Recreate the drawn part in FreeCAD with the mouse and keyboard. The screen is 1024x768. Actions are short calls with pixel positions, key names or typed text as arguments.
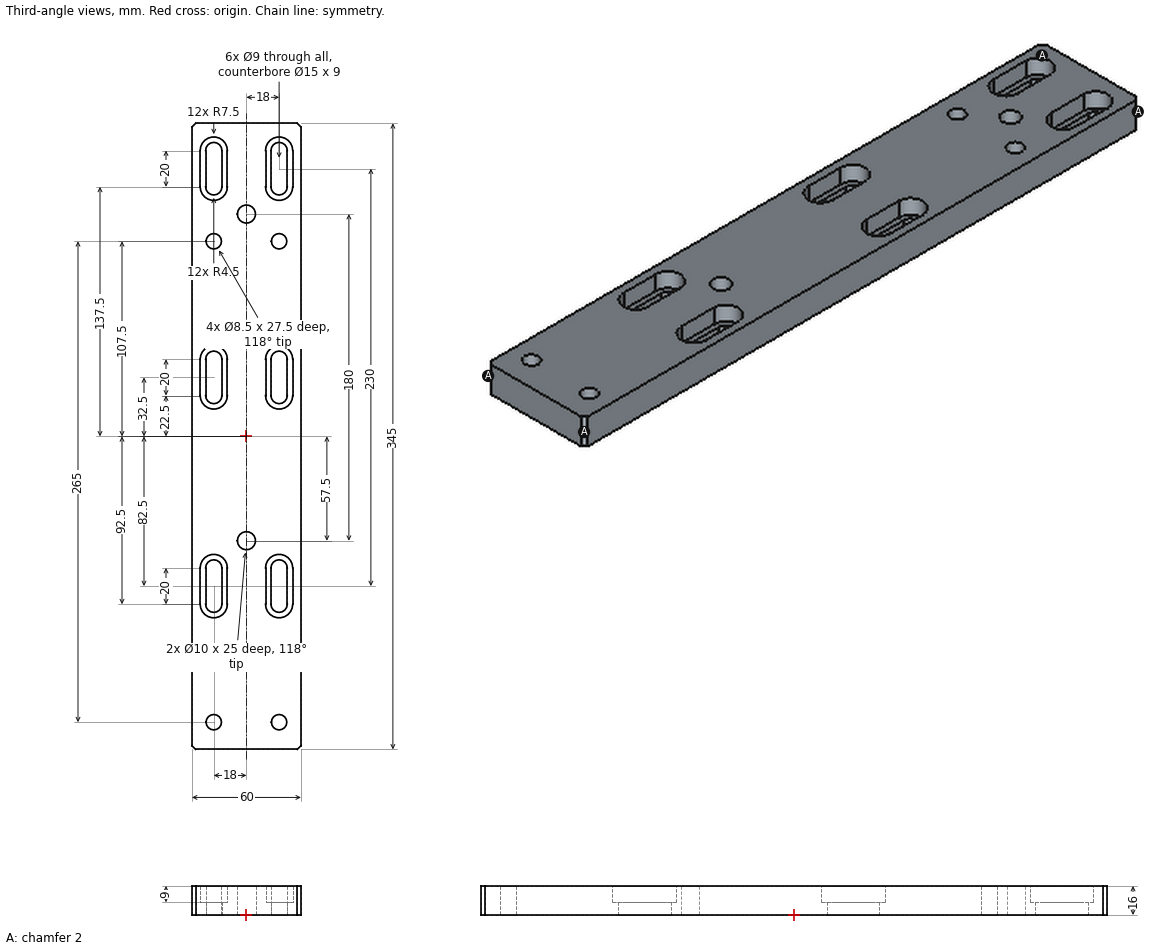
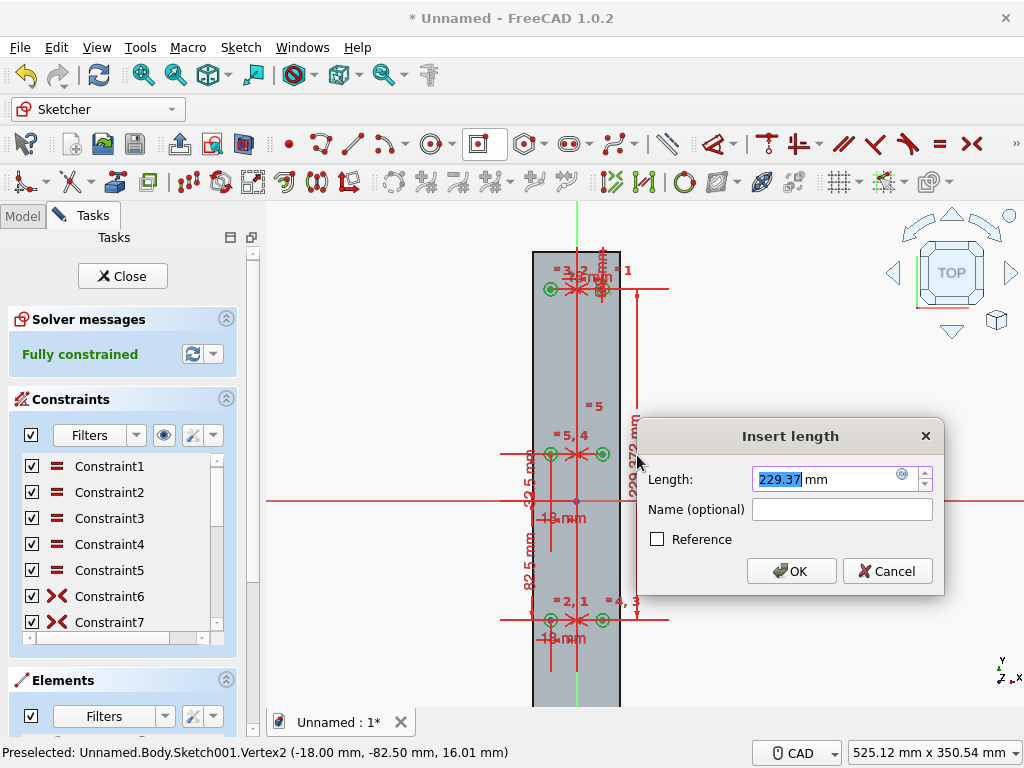
text(230)
key(Return)
key(Escape)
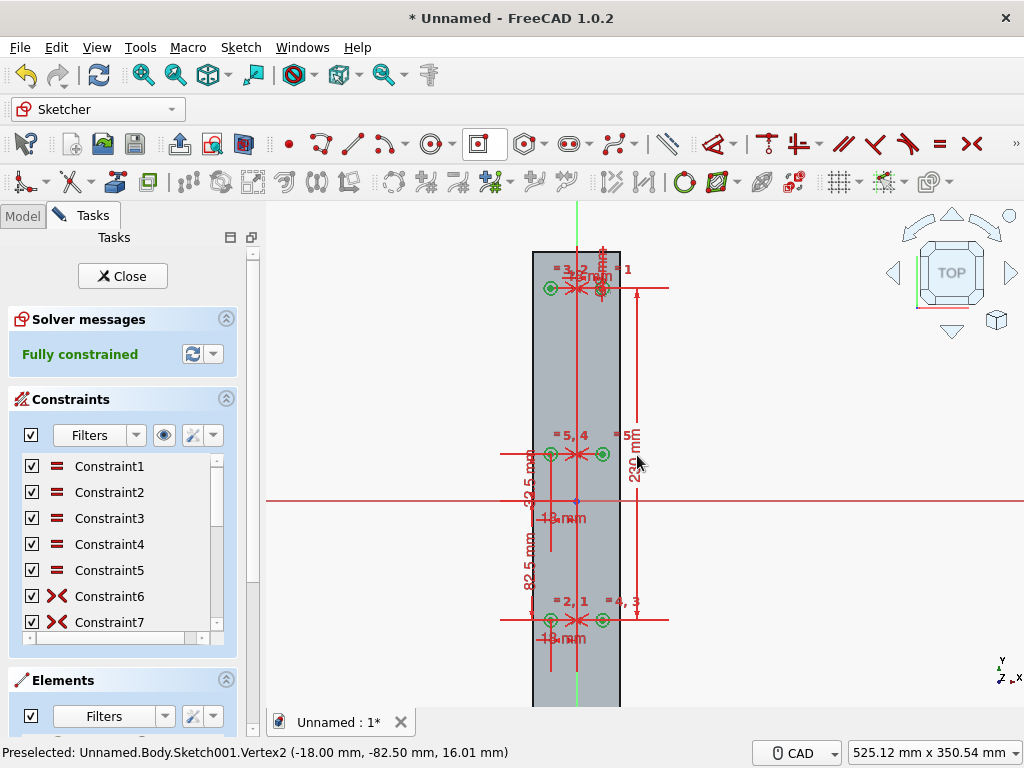
click(123, 276)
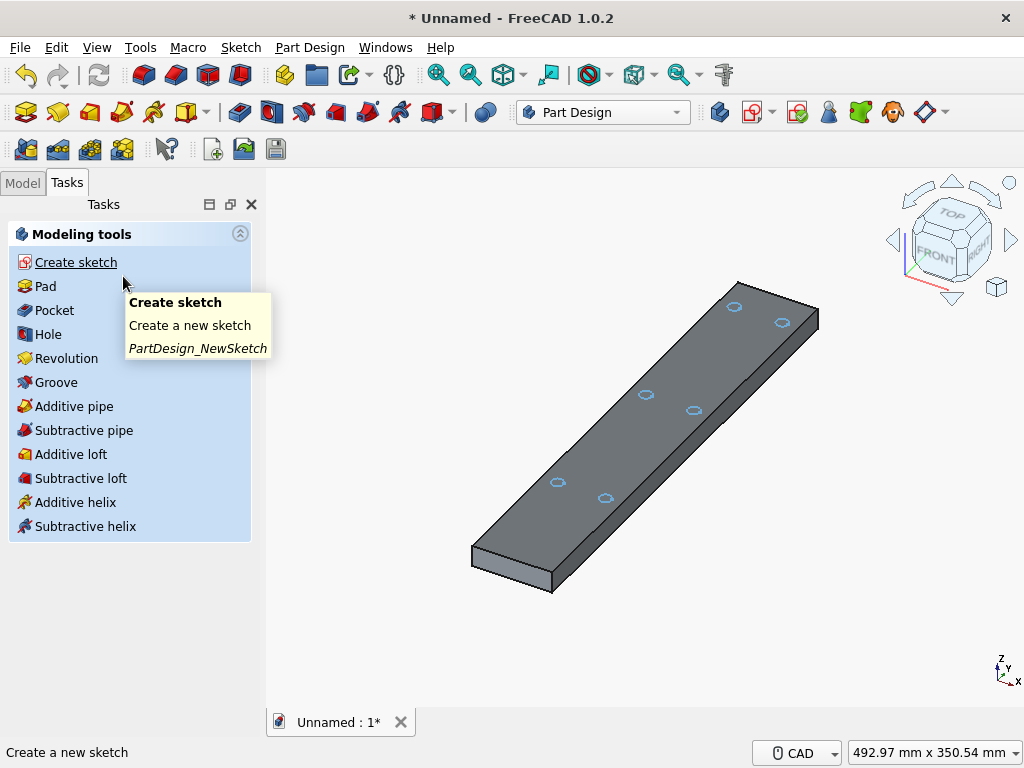
click(272, 112)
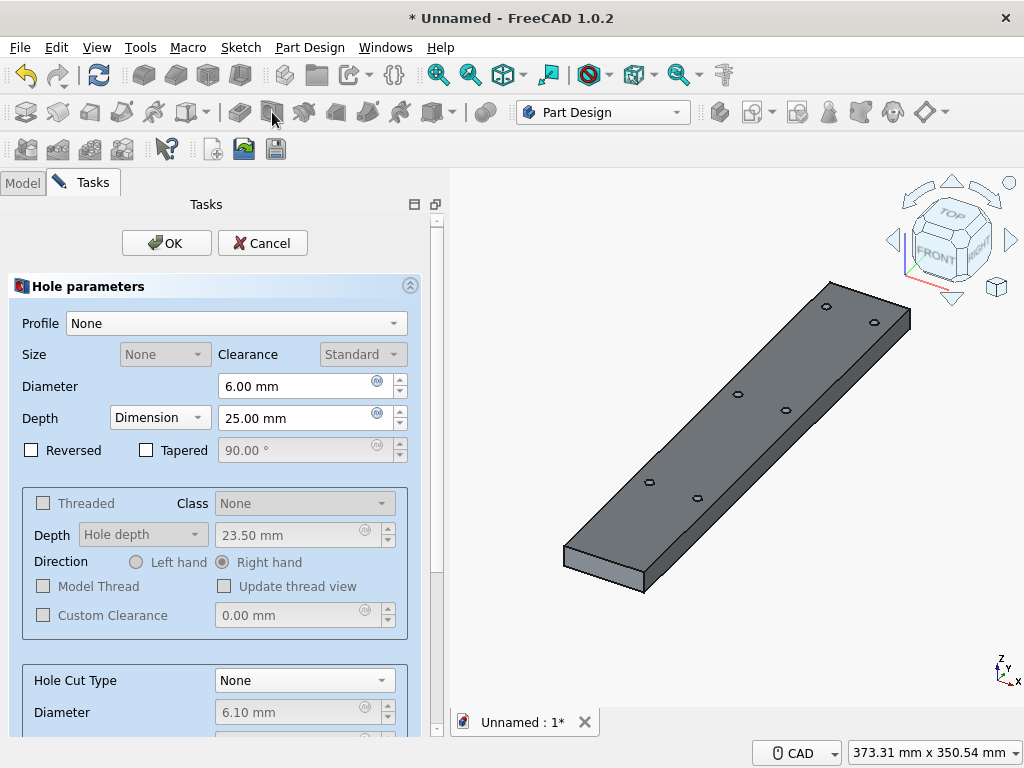
triple_click(305, 386)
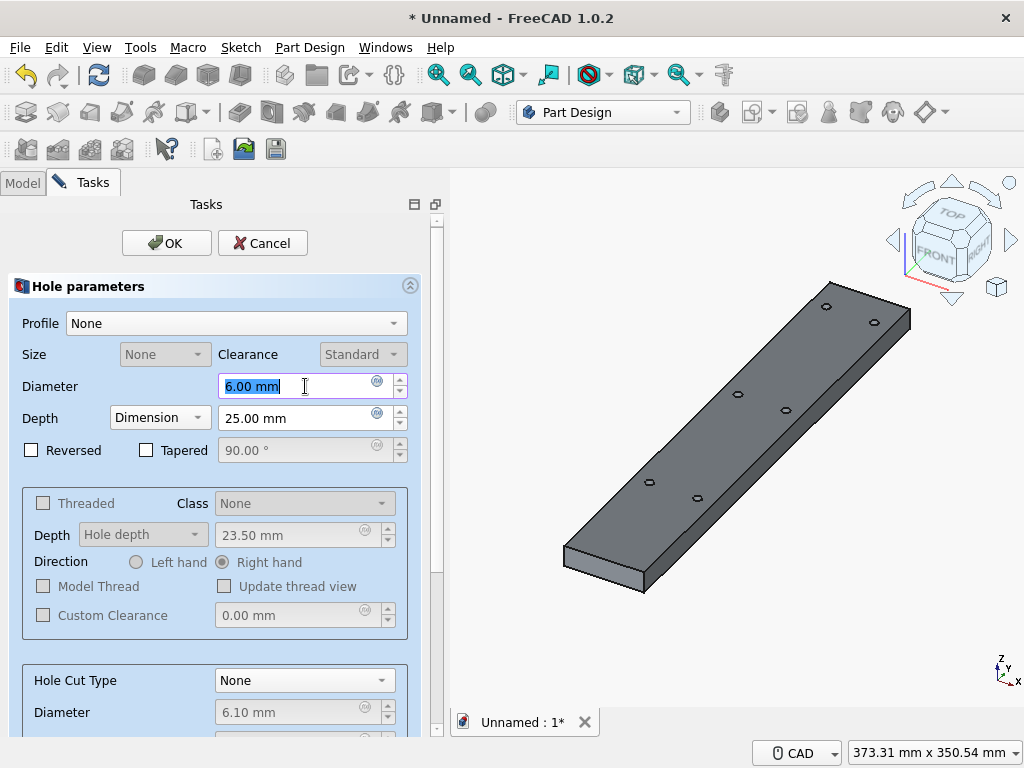
text(9)
key(Tab)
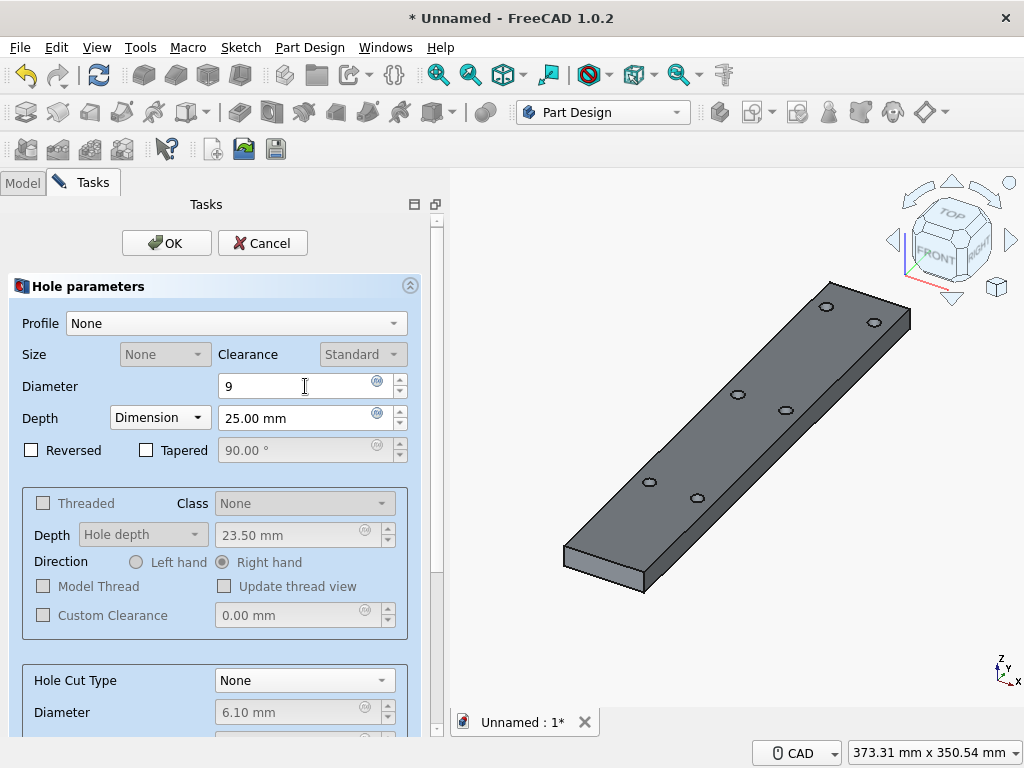
click(161, 418)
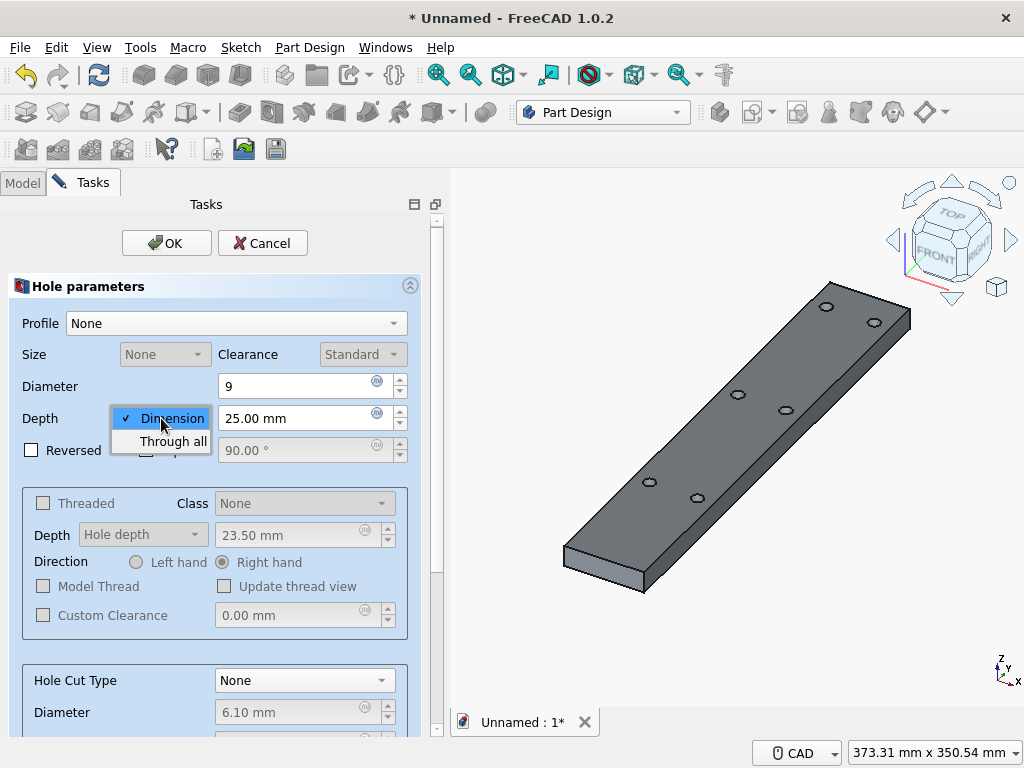
click(160, 442)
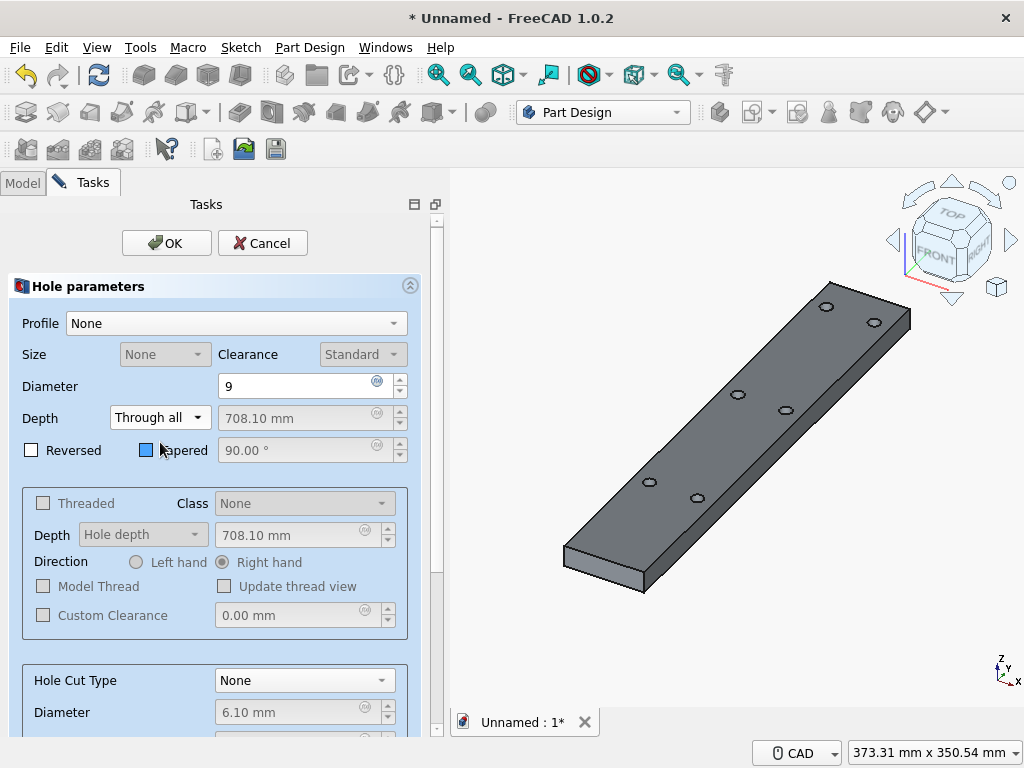
click(306, 680)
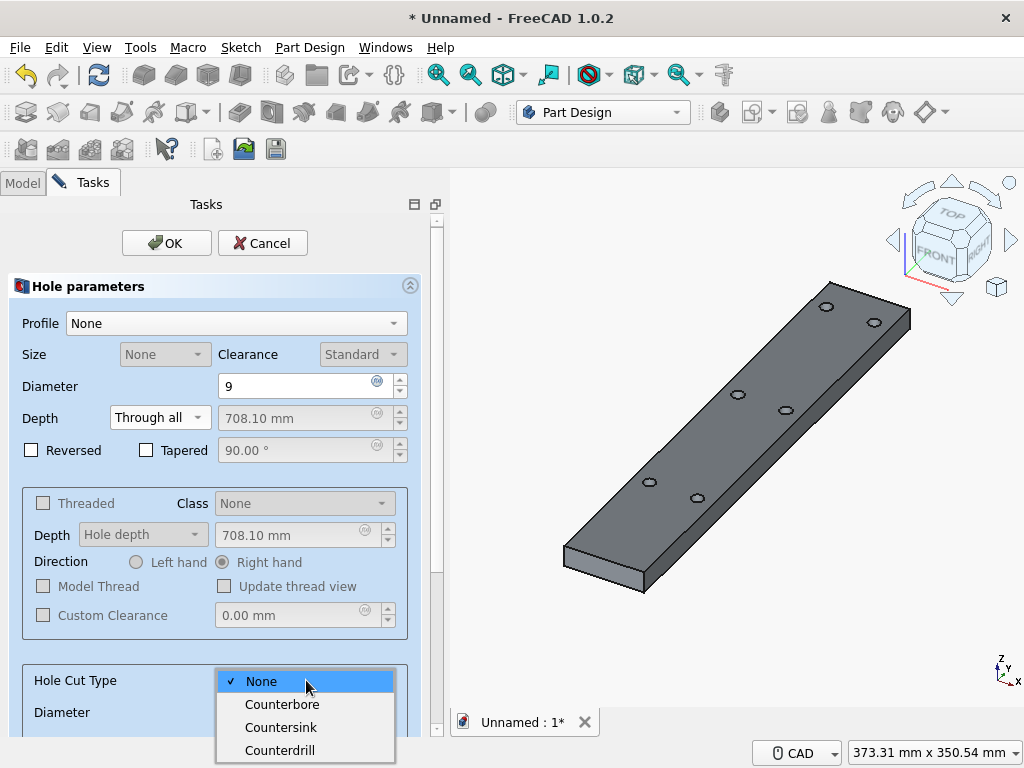
click(304, 704)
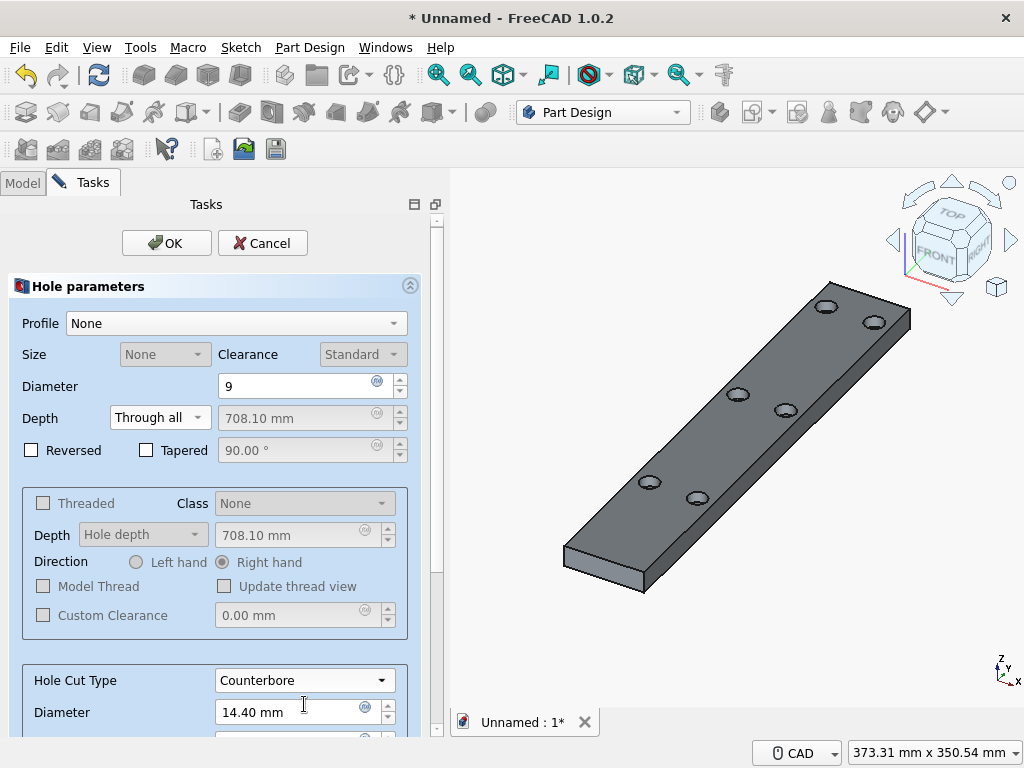
triple_click(298, 712)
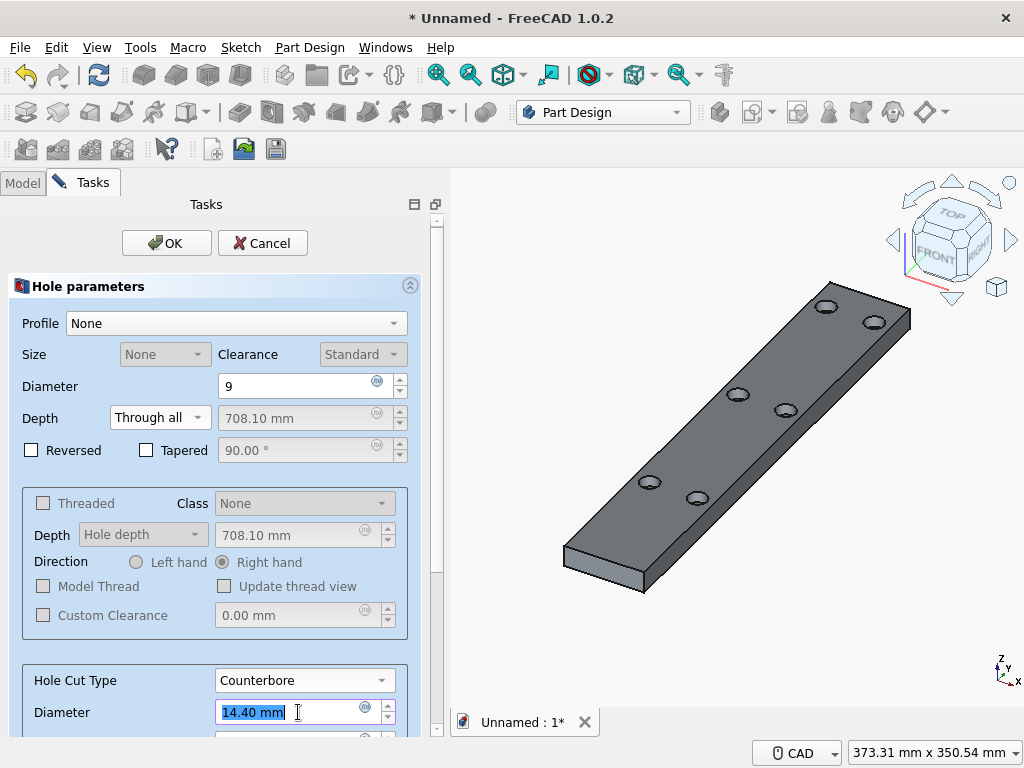
text(15)
key(Tab)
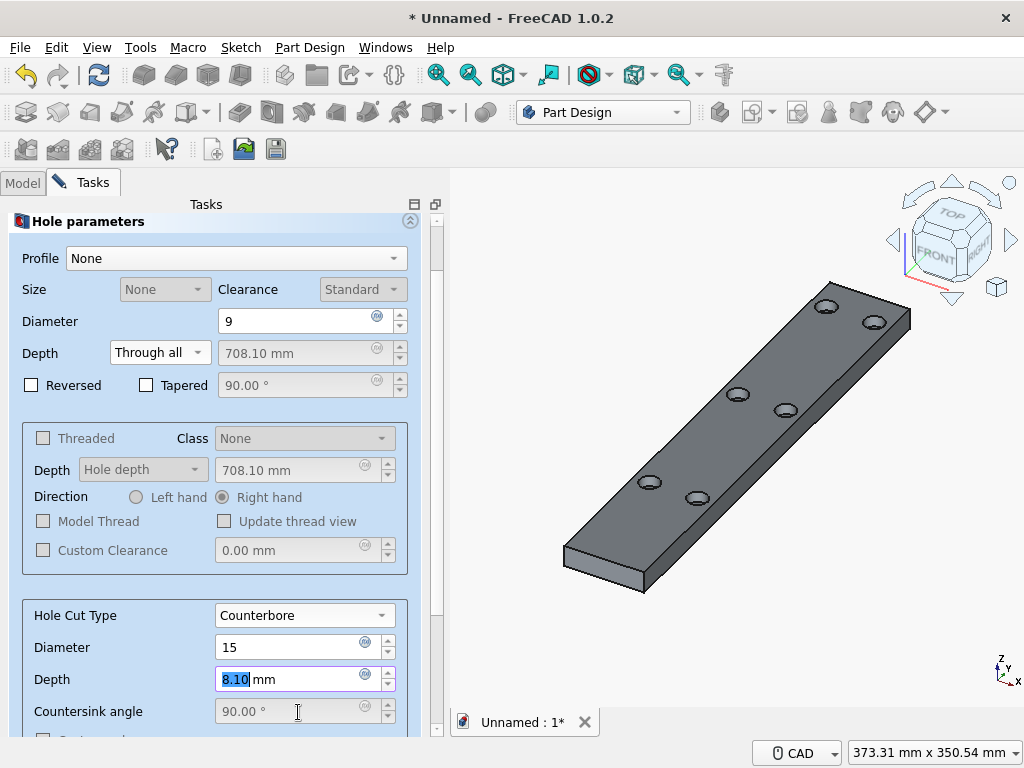
text(9)
key(Tab)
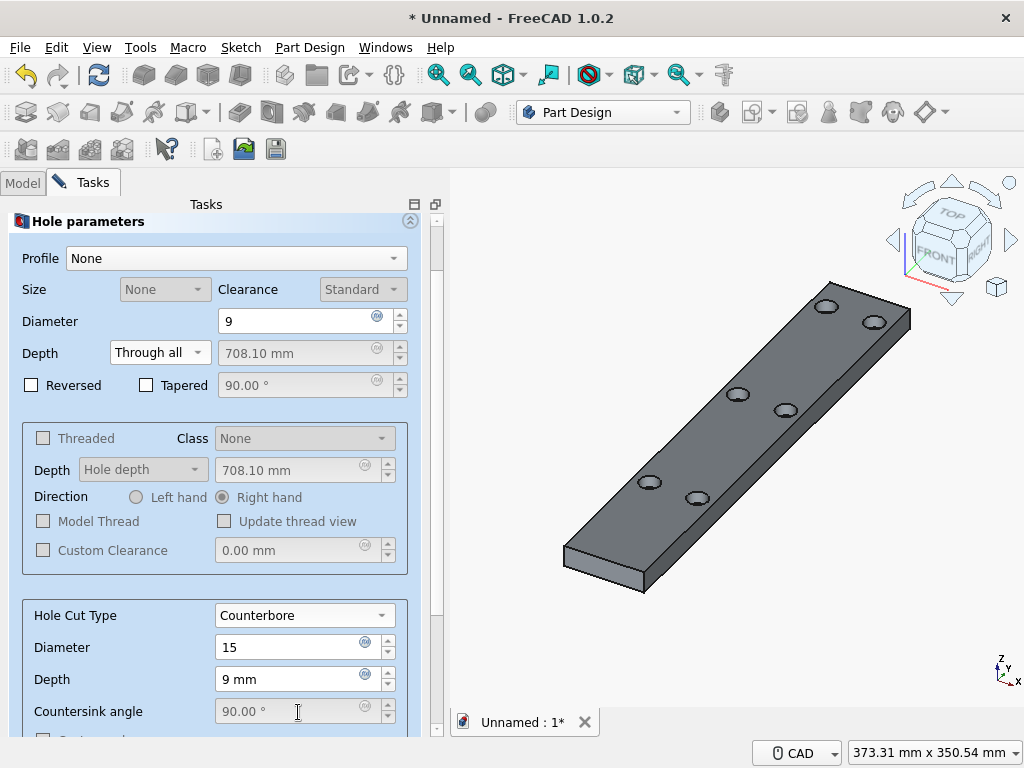
scroll(437, 475, up, 2)